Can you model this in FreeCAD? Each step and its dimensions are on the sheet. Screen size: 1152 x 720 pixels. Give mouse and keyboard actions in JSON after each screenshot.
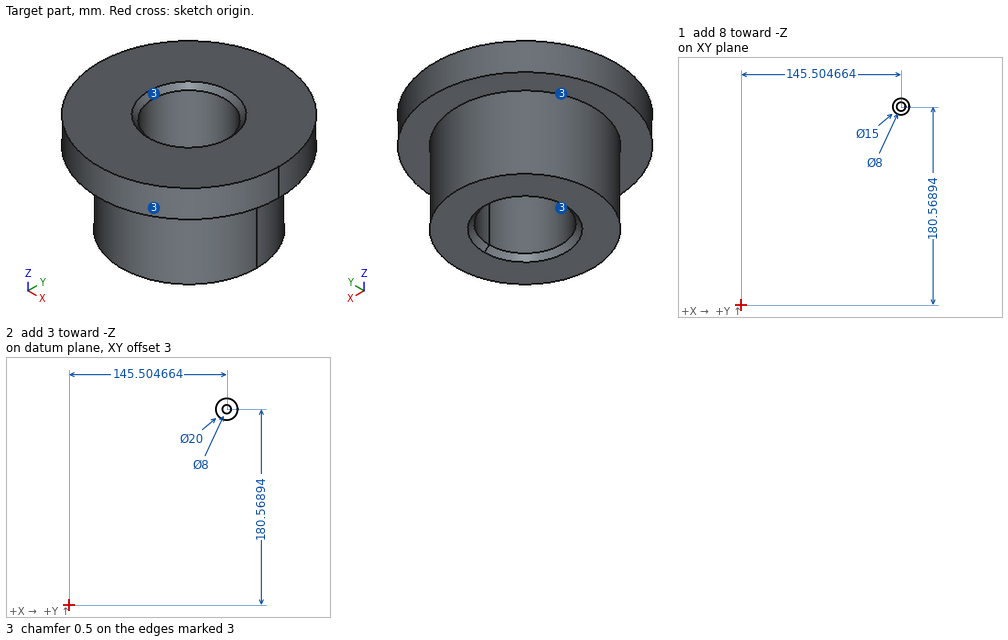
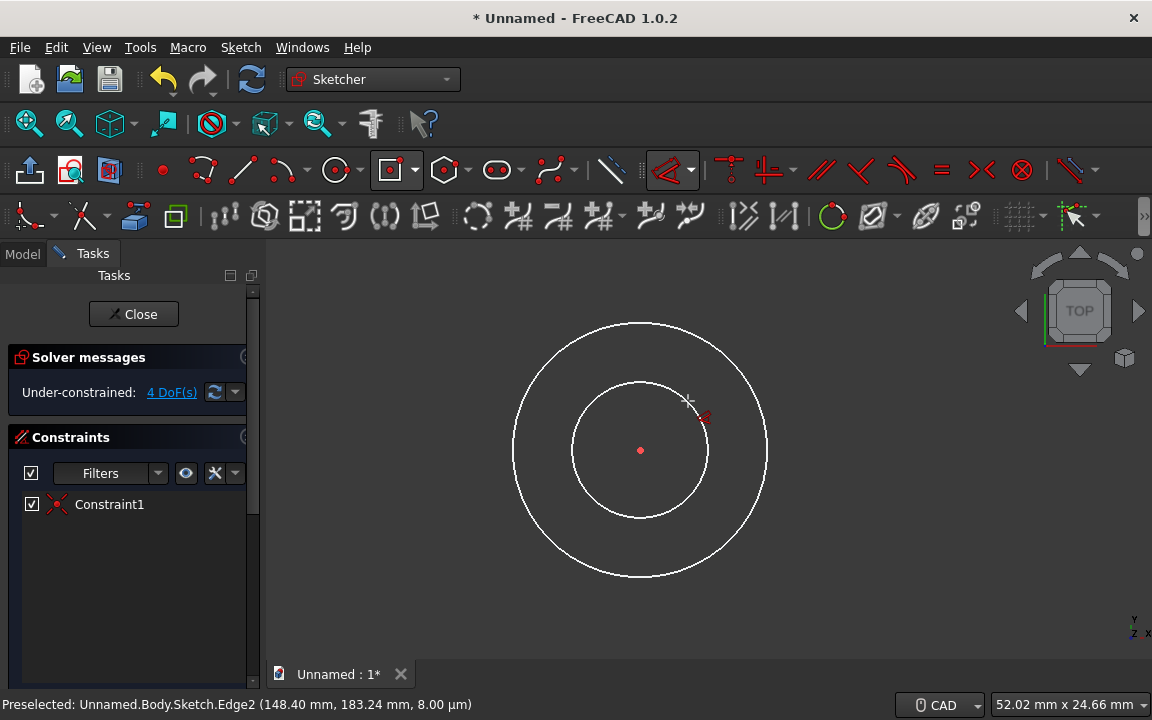
{"action": "left_click", "coordinate": [730, 360]}
{"action": "left_click", "coordinate": [753, 337]}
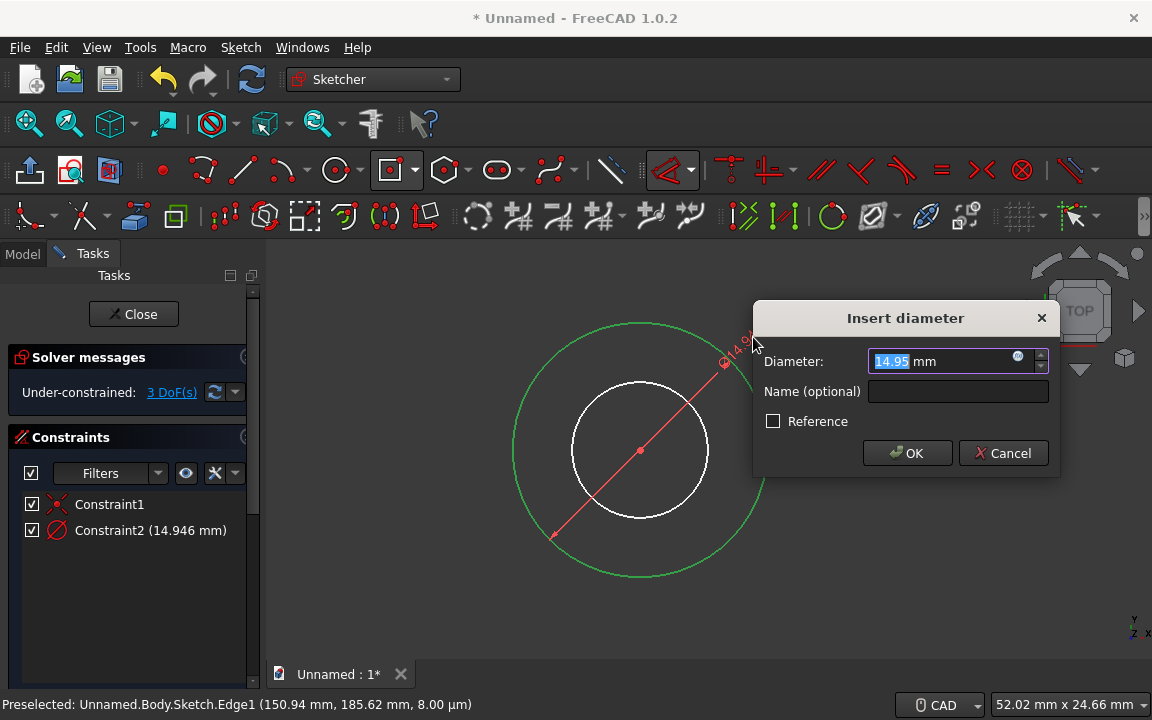
{"action": "type", "text": "15"}
{"action": "key", "text": "Return"}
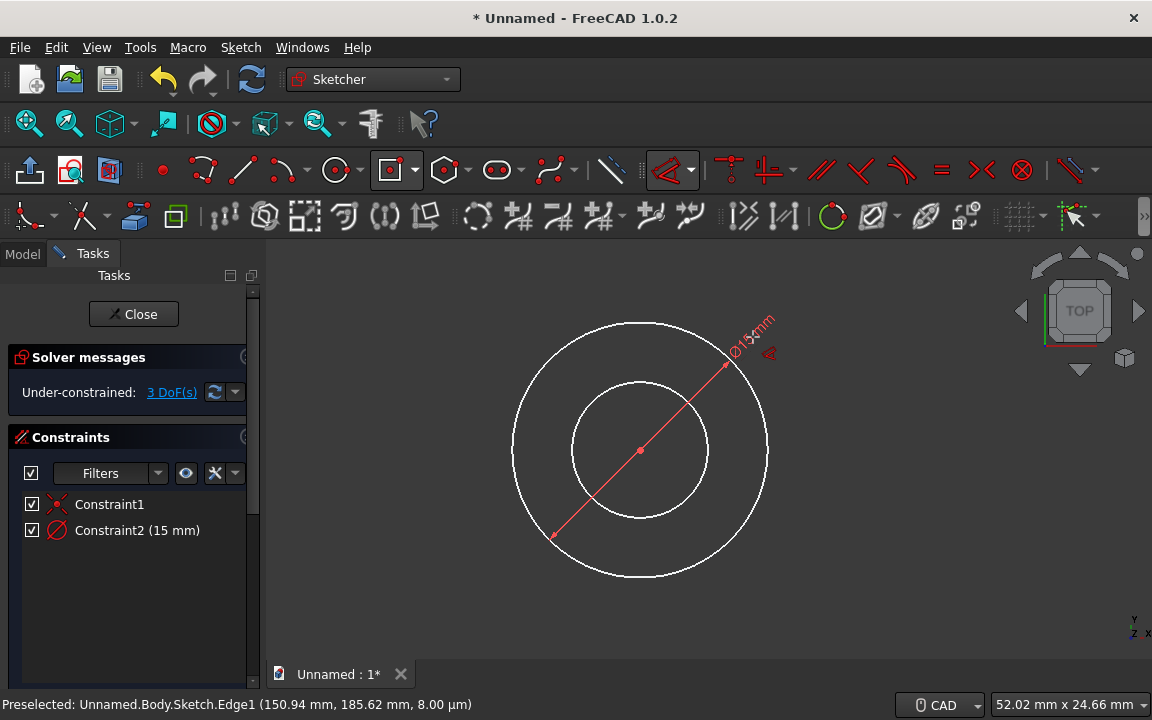
{"action": "left_click", "coordinate": [688, 402]}
{"action": "left_click", "coordinate": [711, 379]}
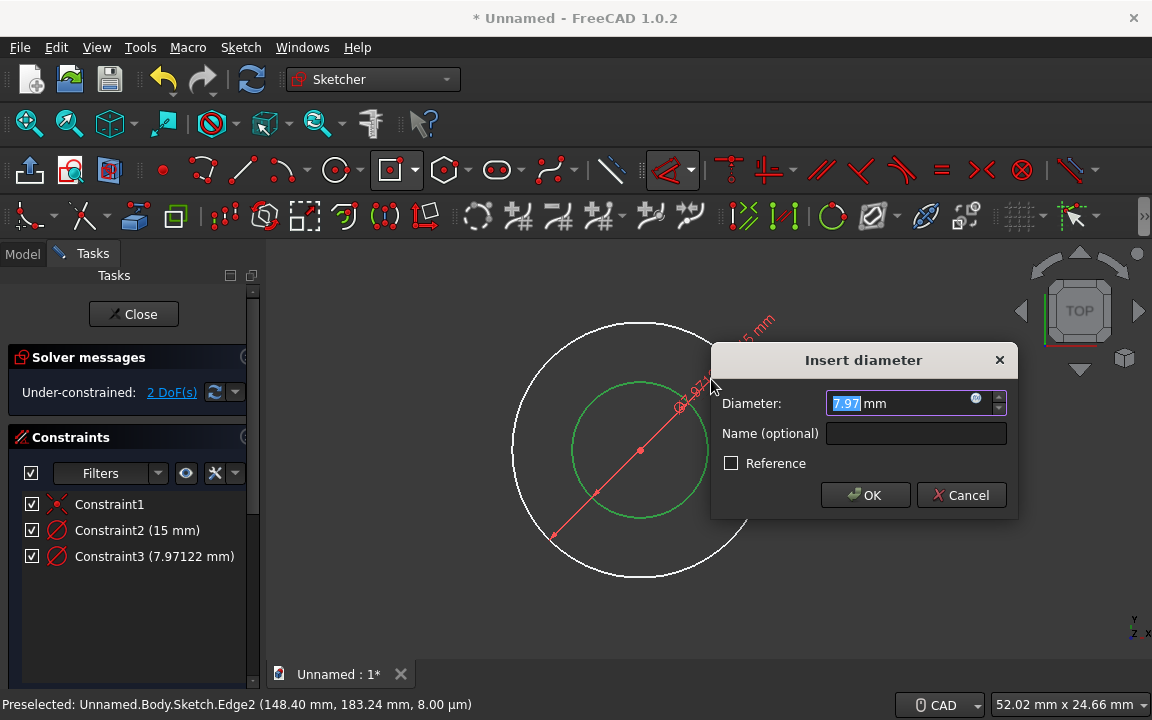
{"action": "type", "text": "8"}
{"action": "key", "text": "Return"}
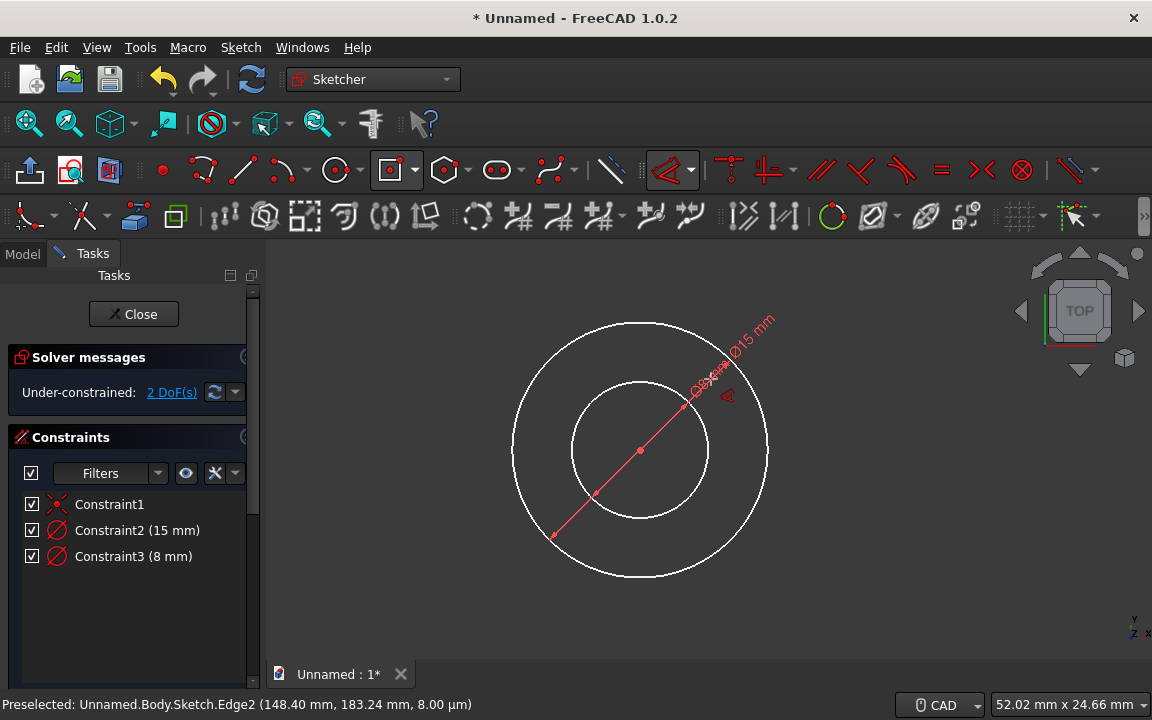
{"action": "left_click", "coordinate": [640, 450]}
{"action": "left_click", "coordinate": [674, 541]}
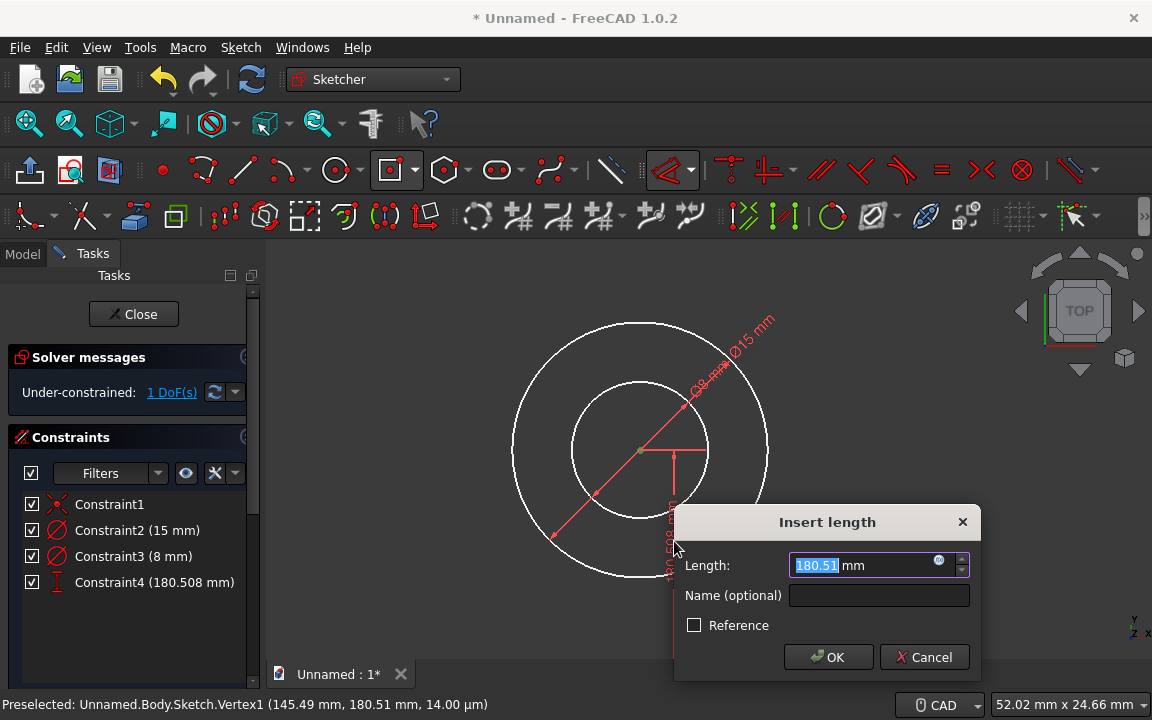
{"action": "type", "text": "180.56894"}
{"action": "key", "text": "Return"}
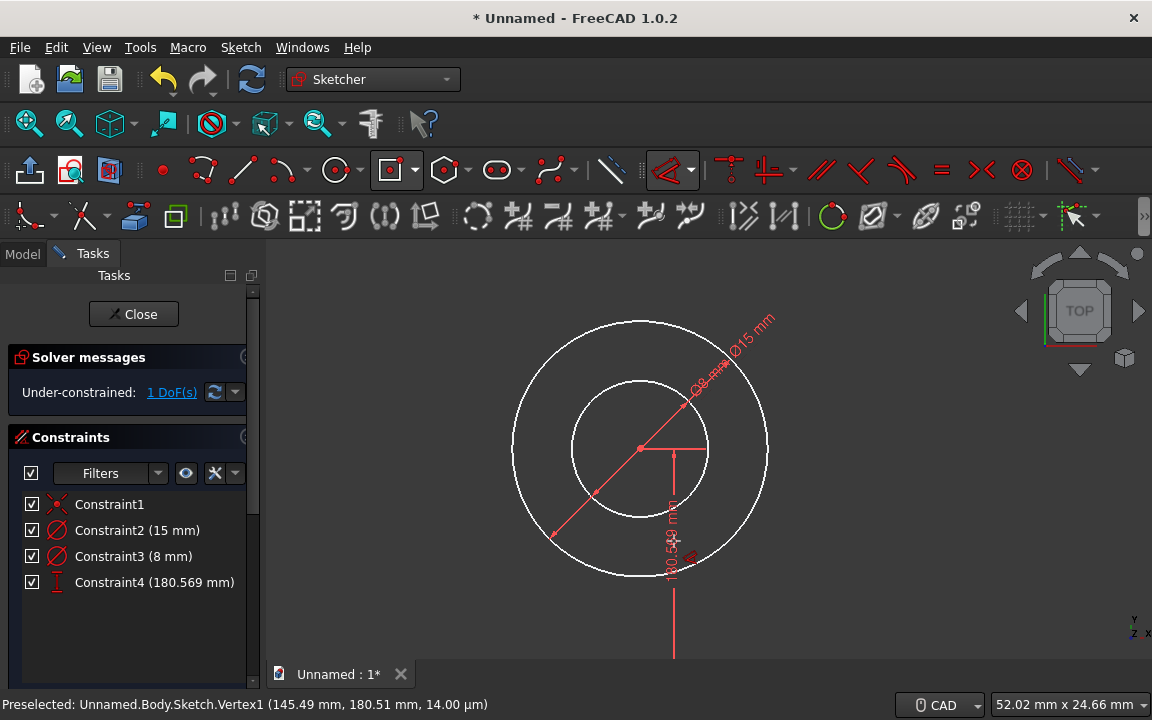
{"action": "left_click", "coordinate": [640, 449]}
{"action": "left_click", "coordinate": [467, 415]}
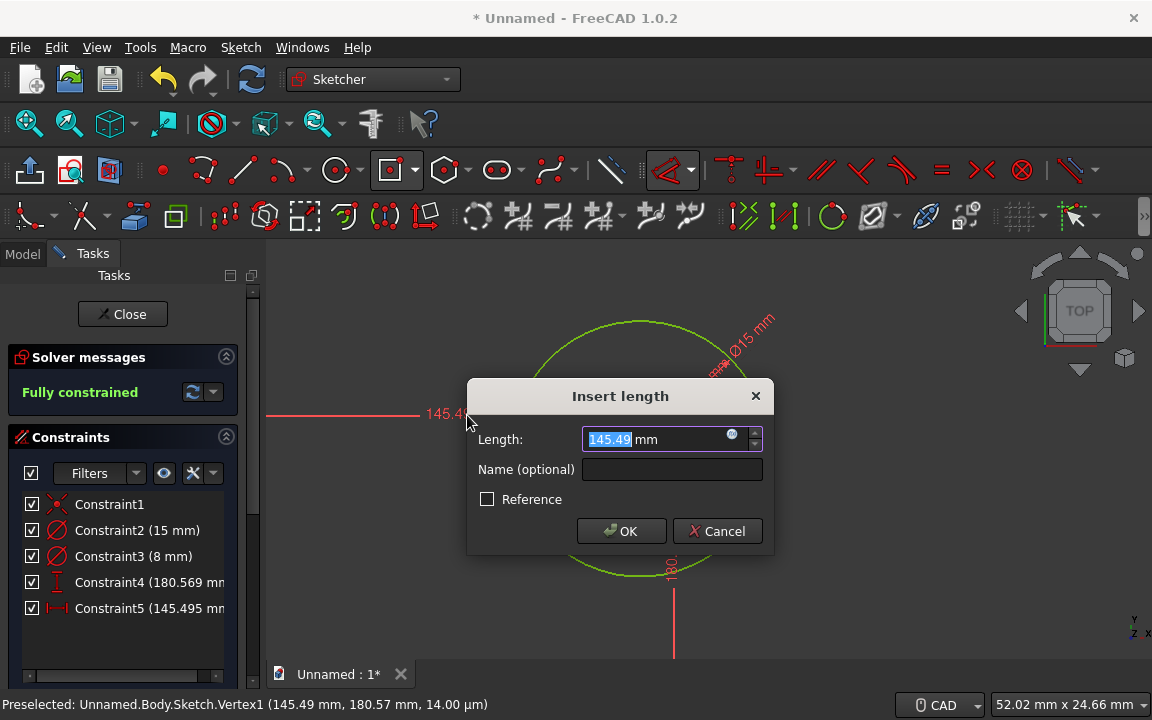
{"action": "type", "text": "145.504664"}
{"action": "key", "text": "Return"}
{"action": "key", "text": "Escape"}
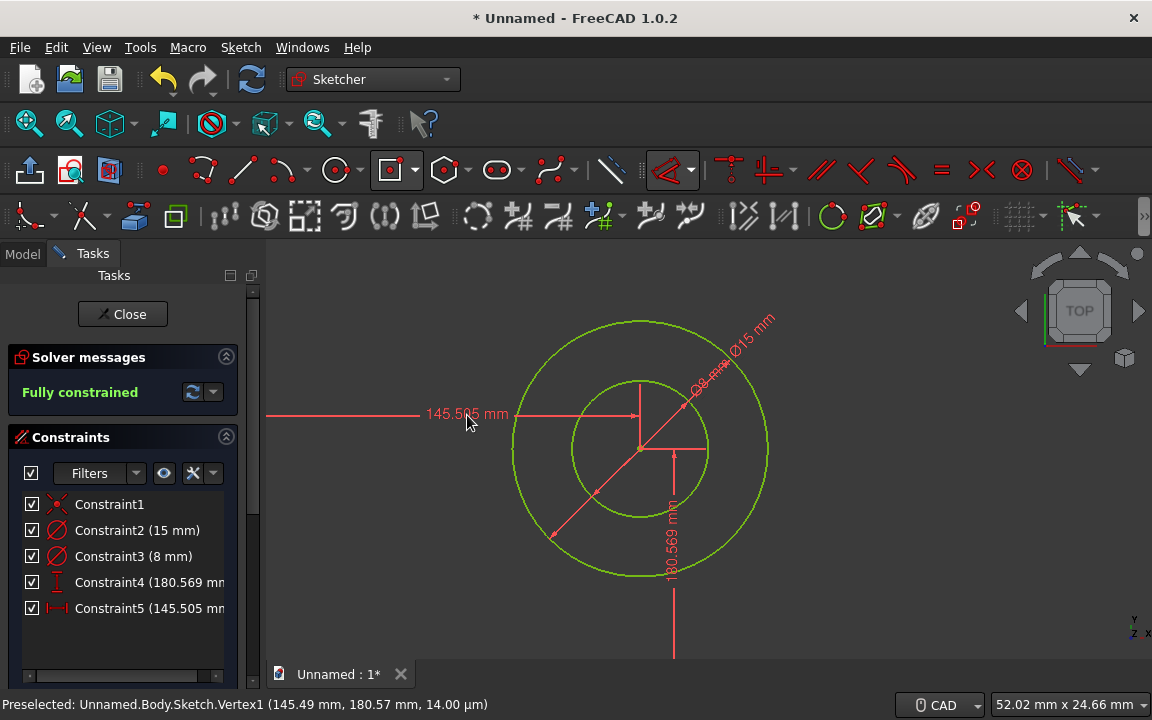
{"action": "left_click", "coordinate": [123, 314]}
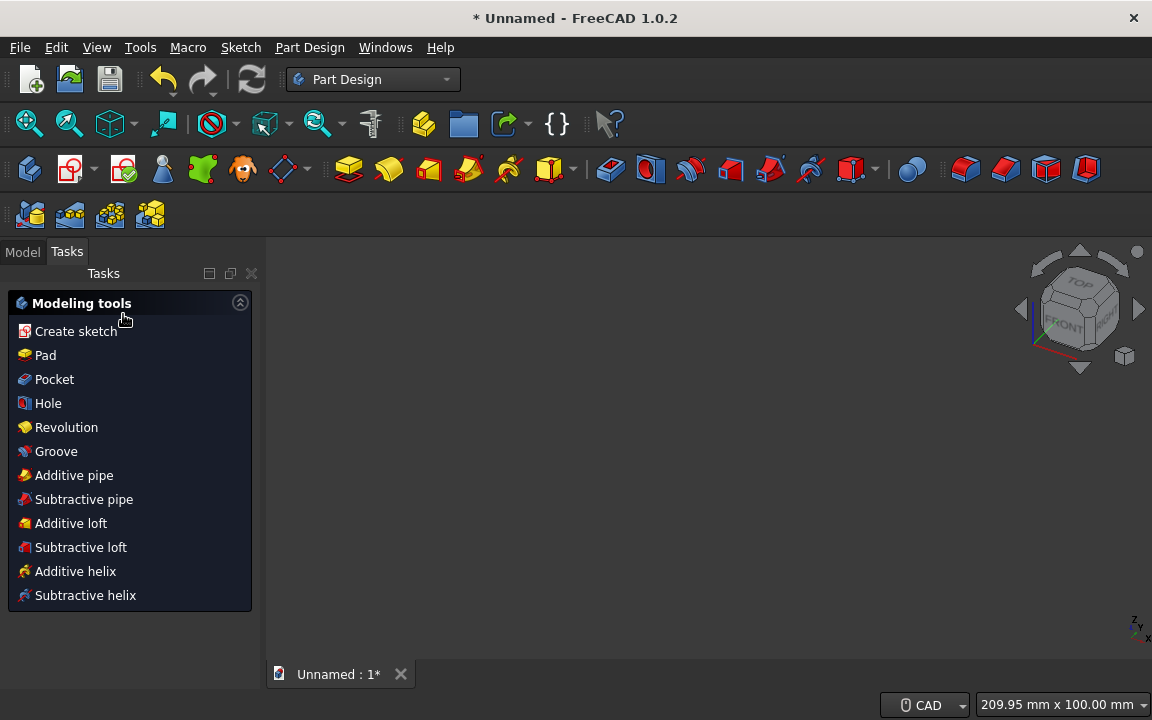
{"action": "left_click", "coordinate": [350, 170]}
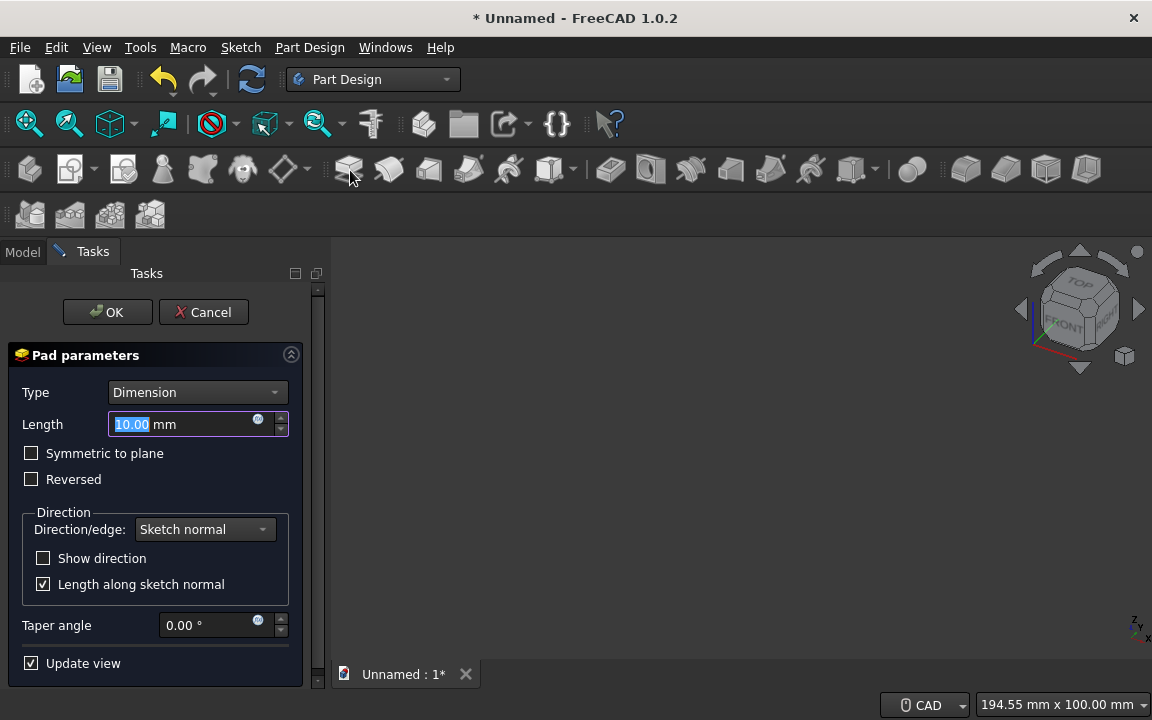
{"action": "type", "text": "8"}
{"action": "key", "text": "Tab"}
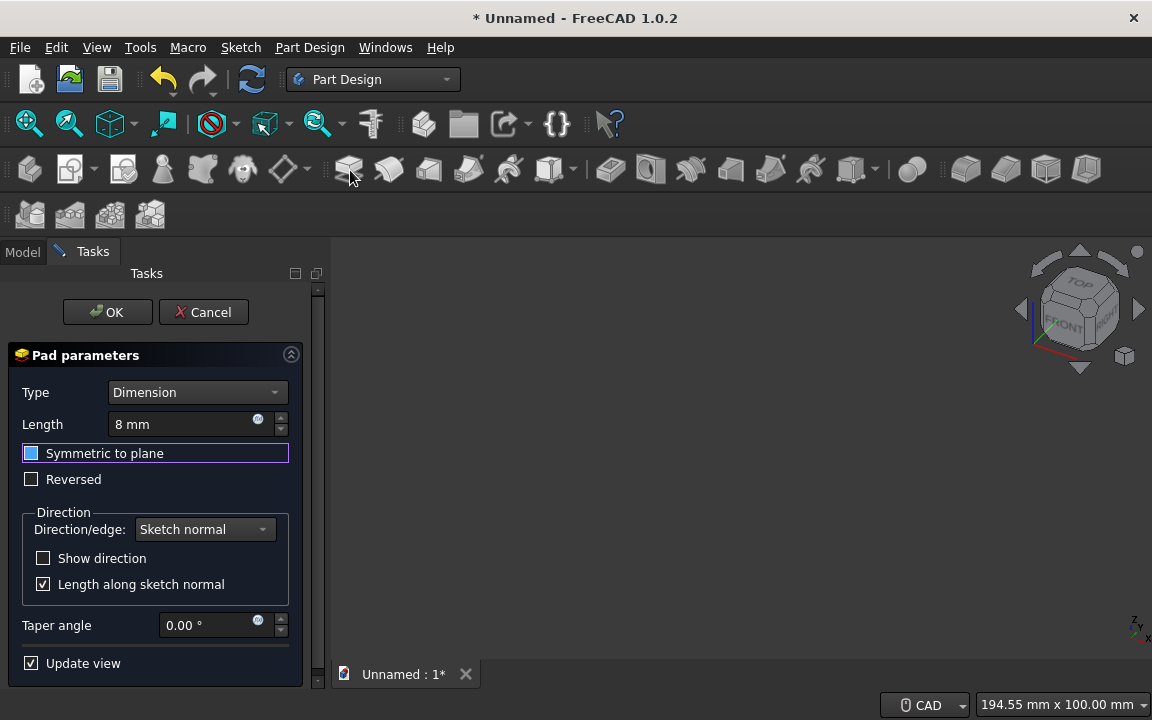
{"action": "left_click", "coordinate": [30, 479]}